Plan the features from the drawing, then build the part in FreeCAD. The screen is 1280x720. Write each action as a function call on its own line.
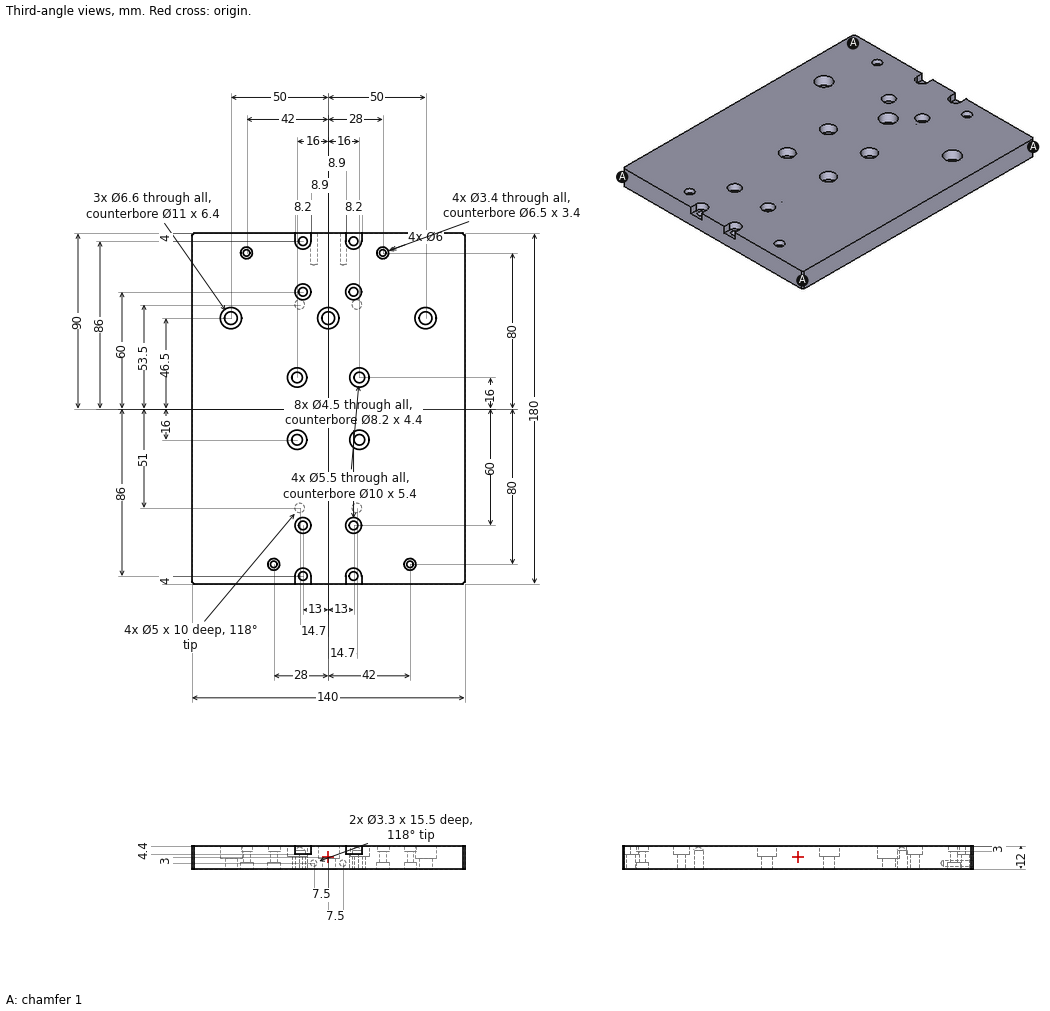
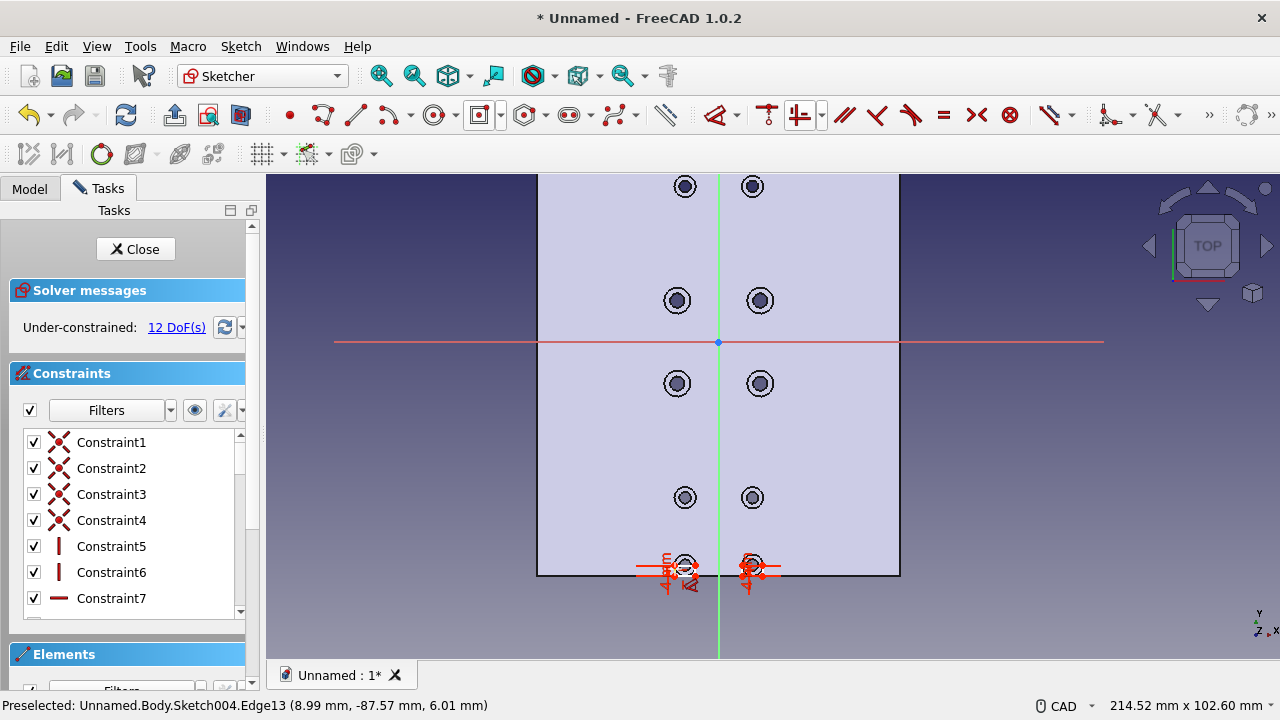
scroll(679, 268, up, 6)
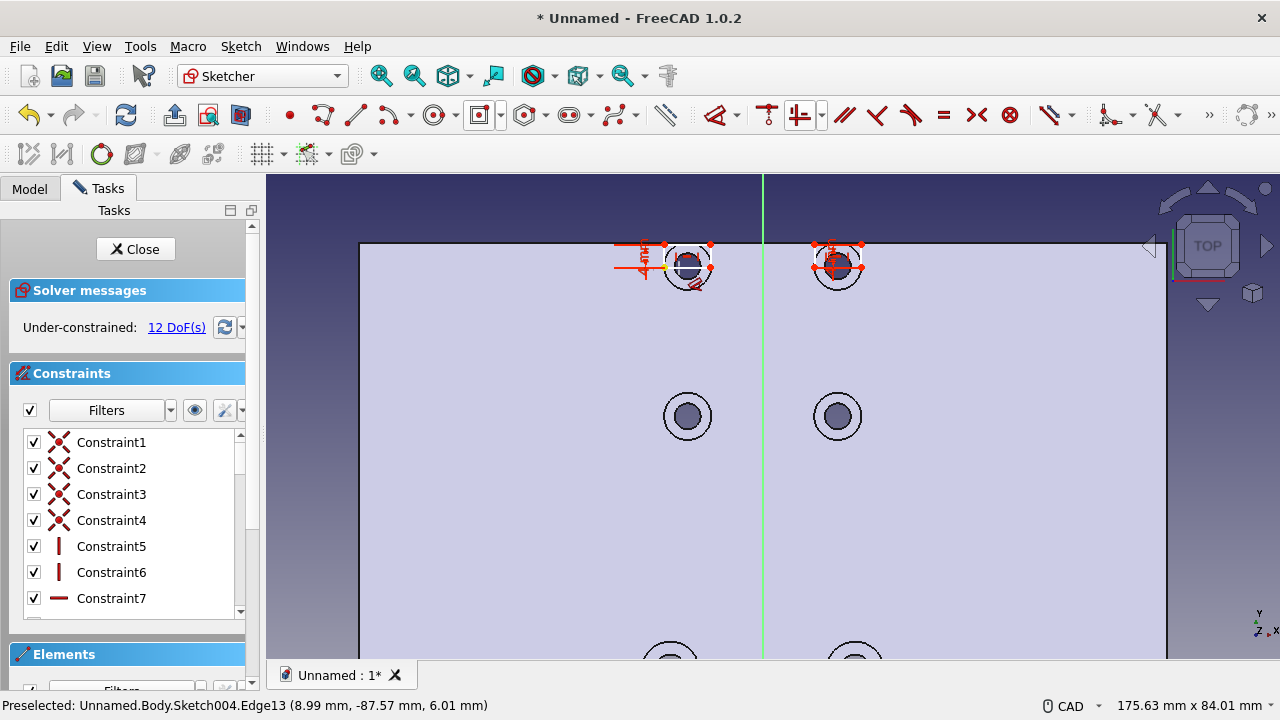
click(678, 268)
click(688, 302)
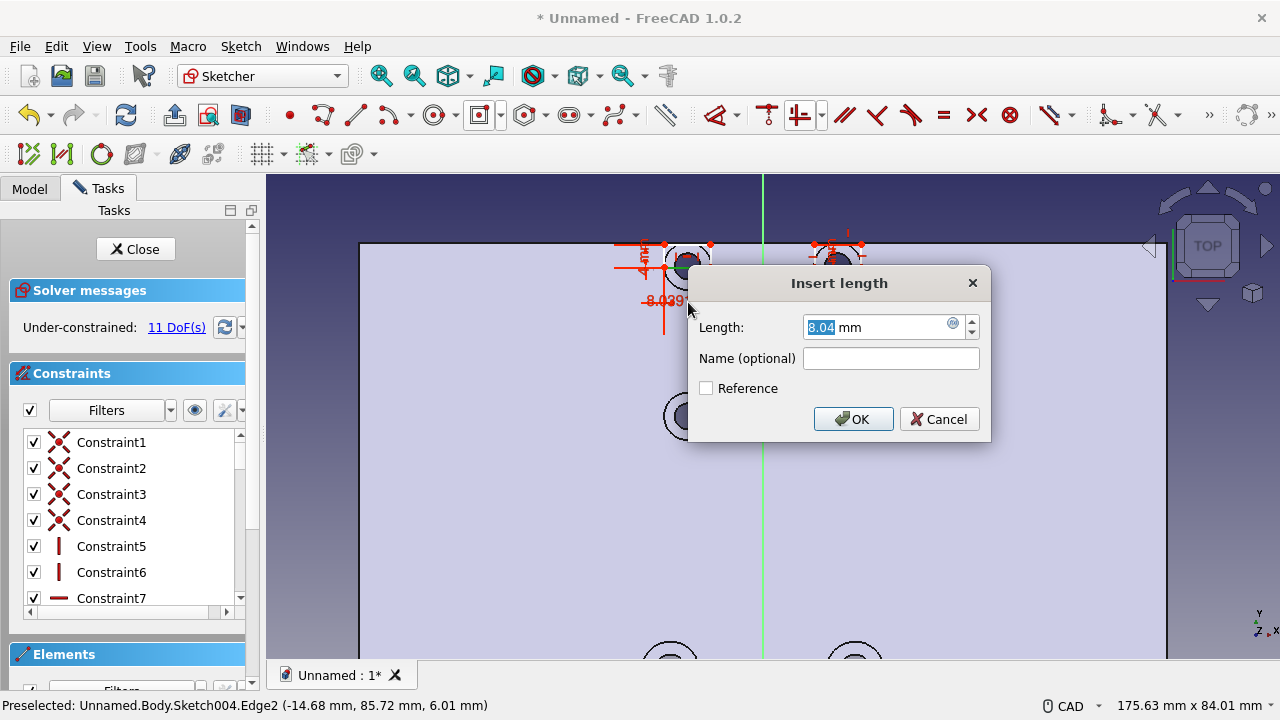
text(8.2)
key(Return)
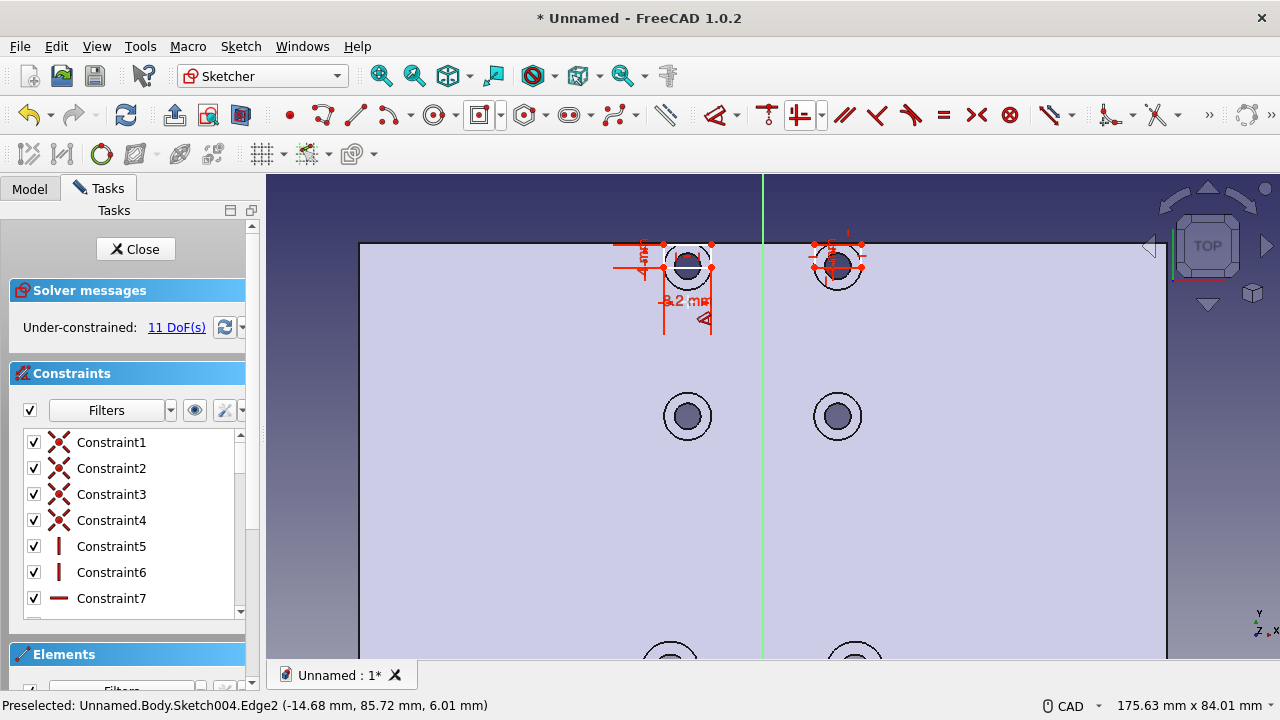
click(829, 268)
click(838, 302)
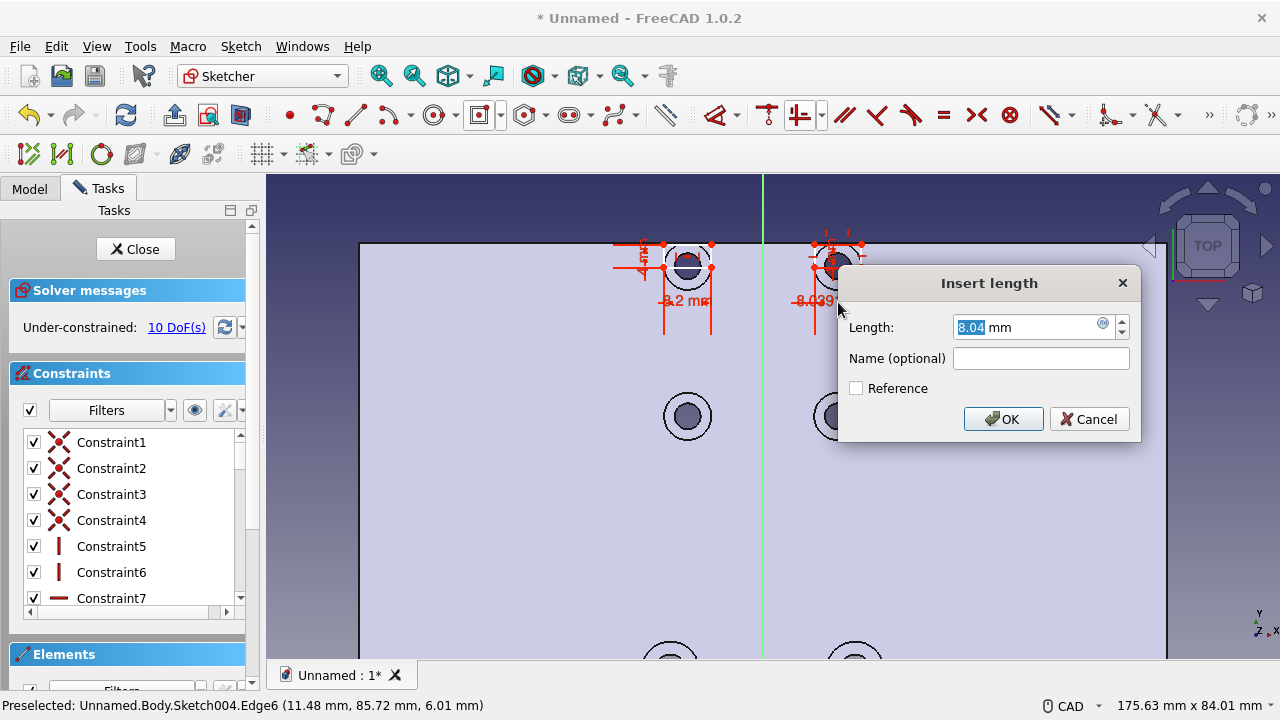
text(8.2)
key(Return)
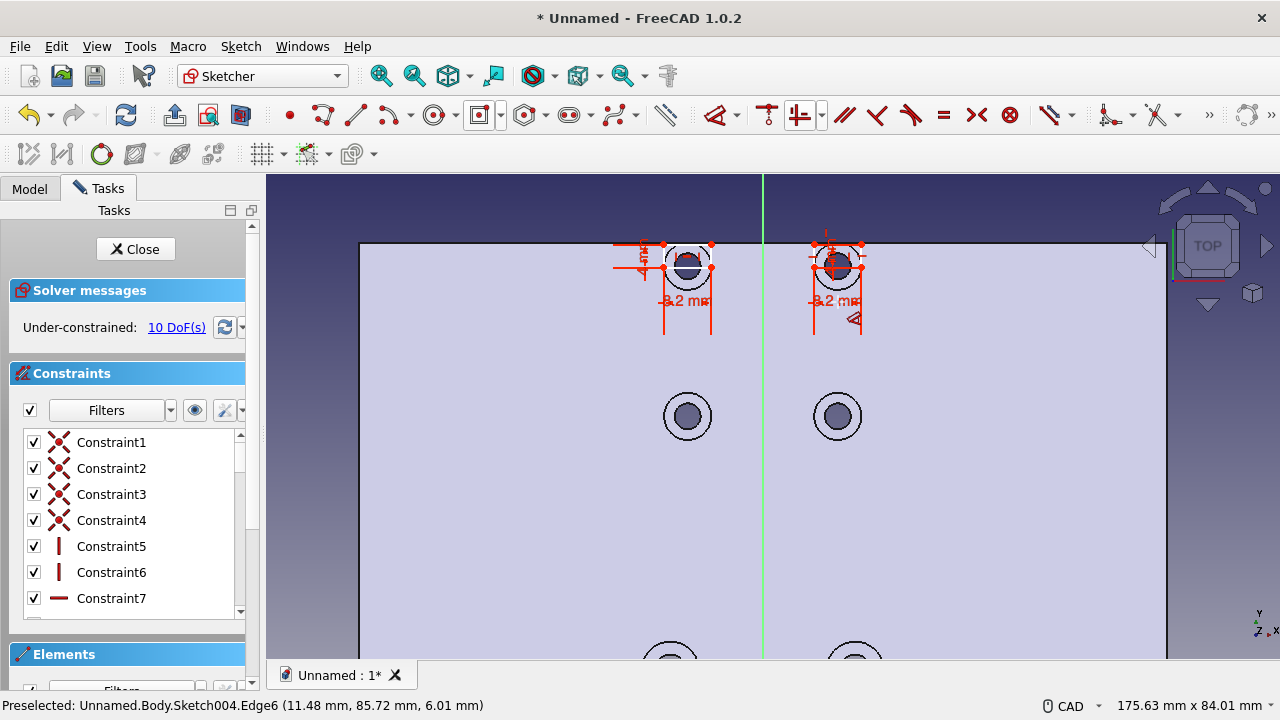
scroll(679, 267, down, 6)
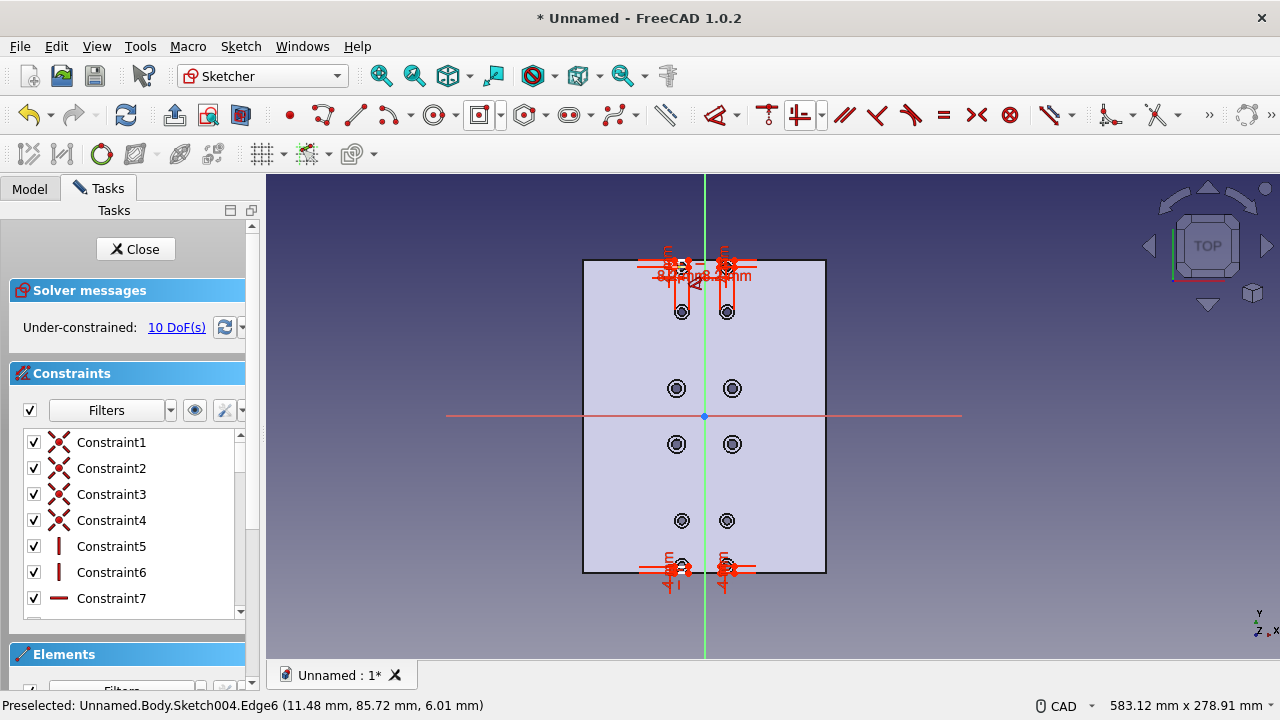
scroll(679, 573, up, 6)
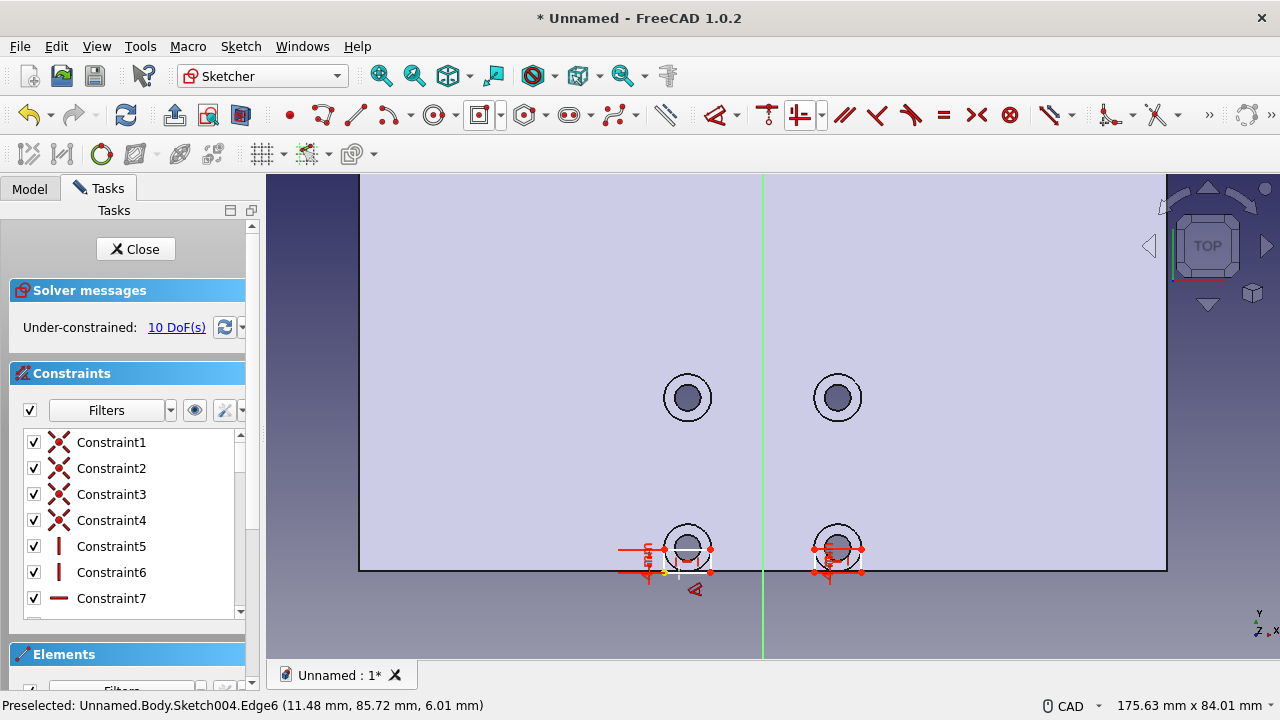
click(678, 573)
click(688, 607)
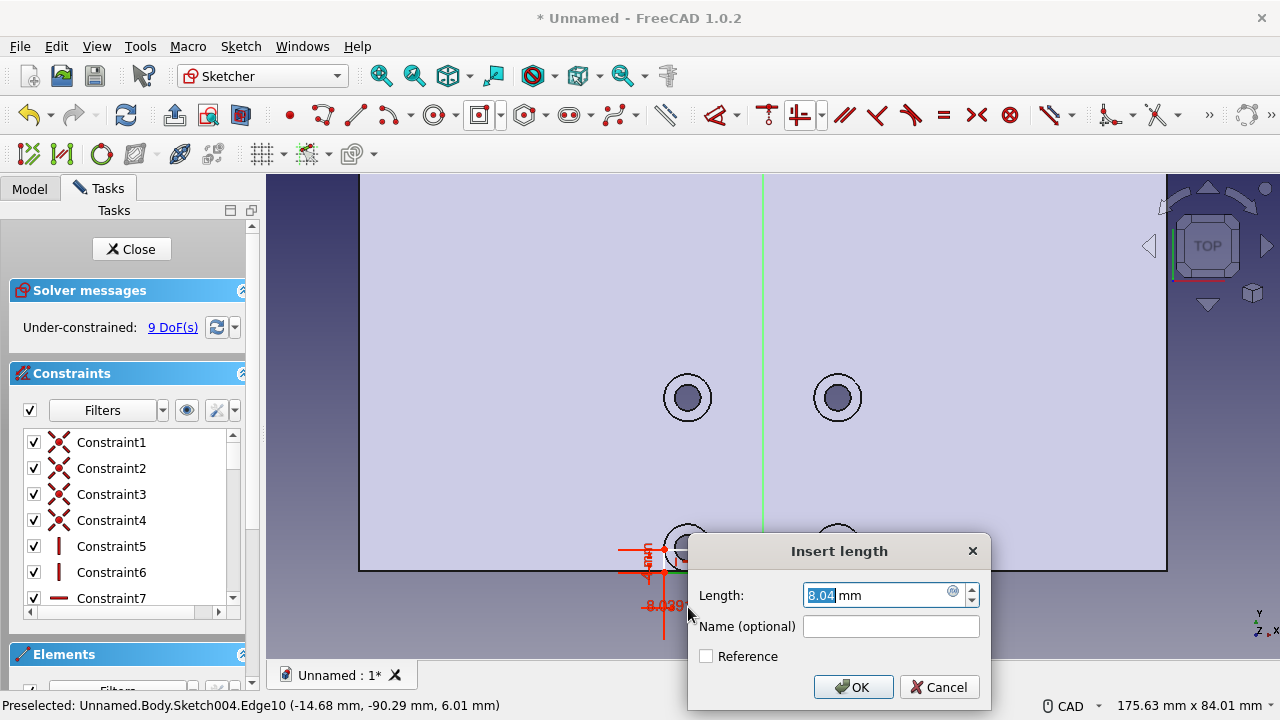
text(8.2)
key(Return)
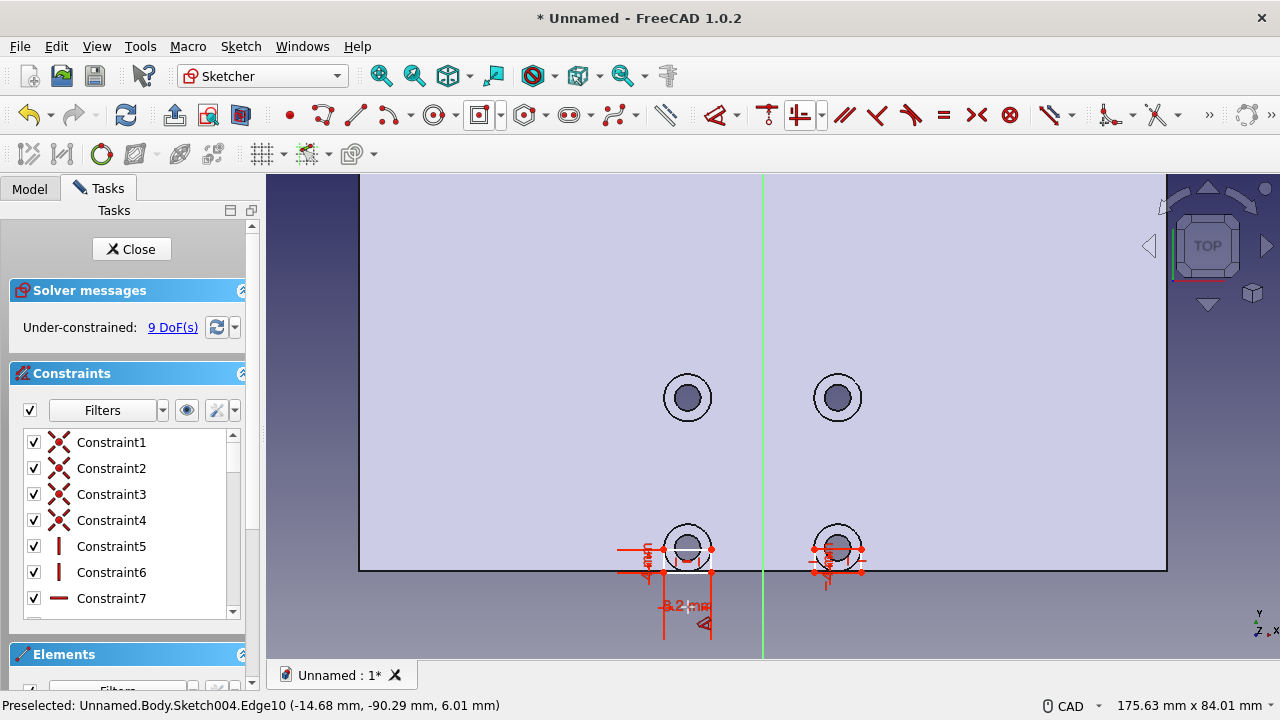
click(829, 573)
click(838, 607)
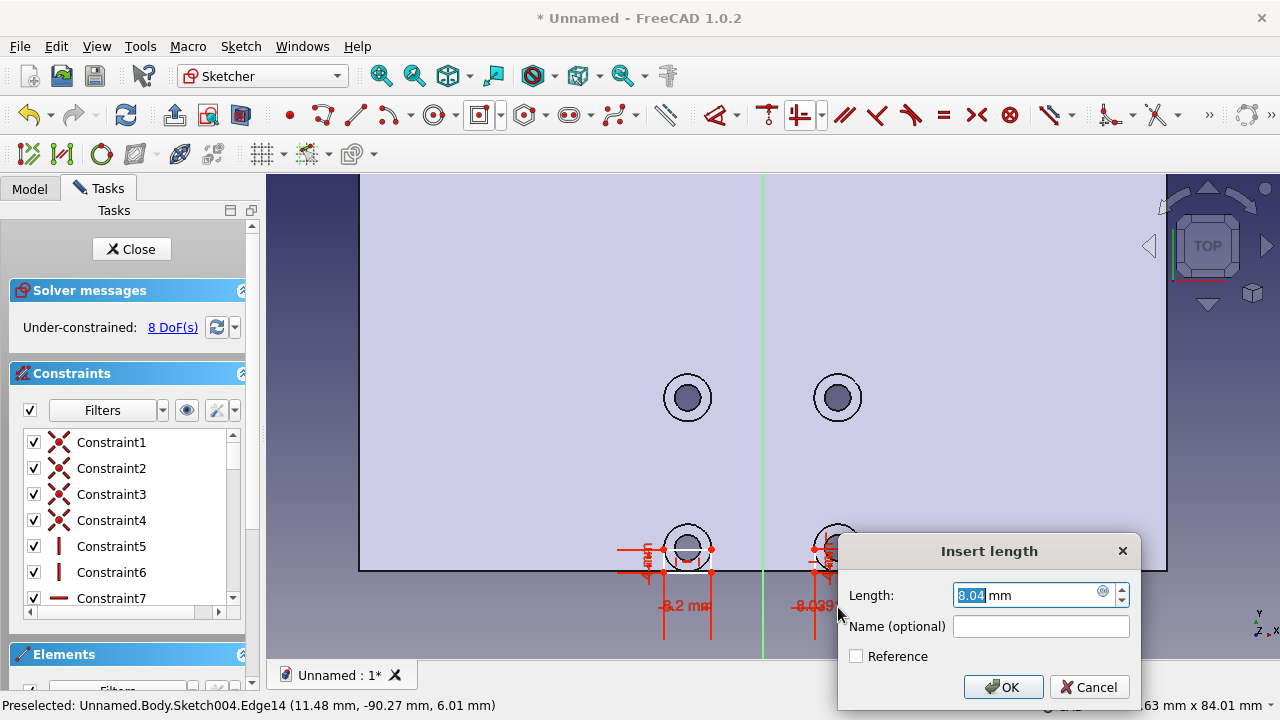
text(8.2)
key(Return)